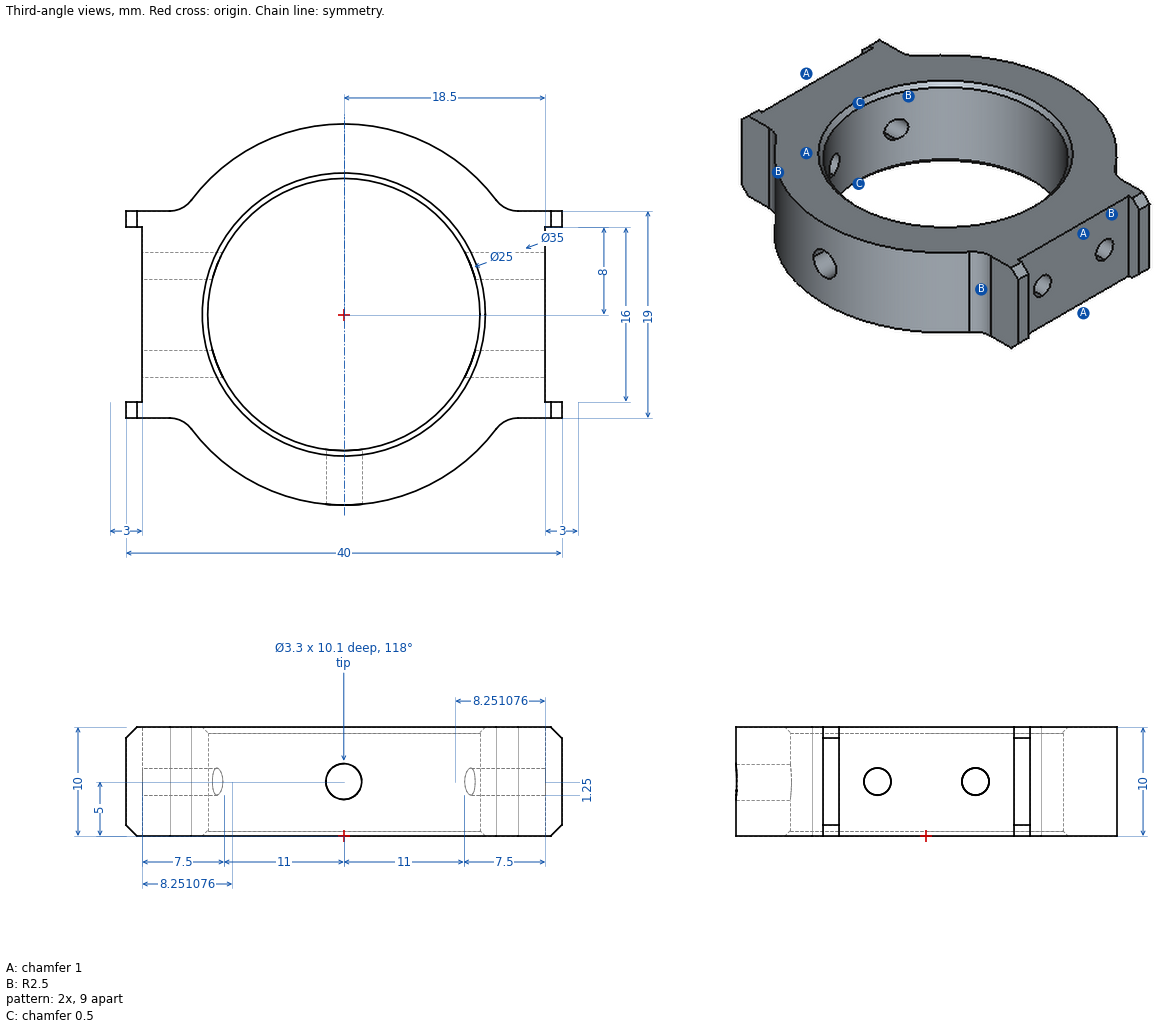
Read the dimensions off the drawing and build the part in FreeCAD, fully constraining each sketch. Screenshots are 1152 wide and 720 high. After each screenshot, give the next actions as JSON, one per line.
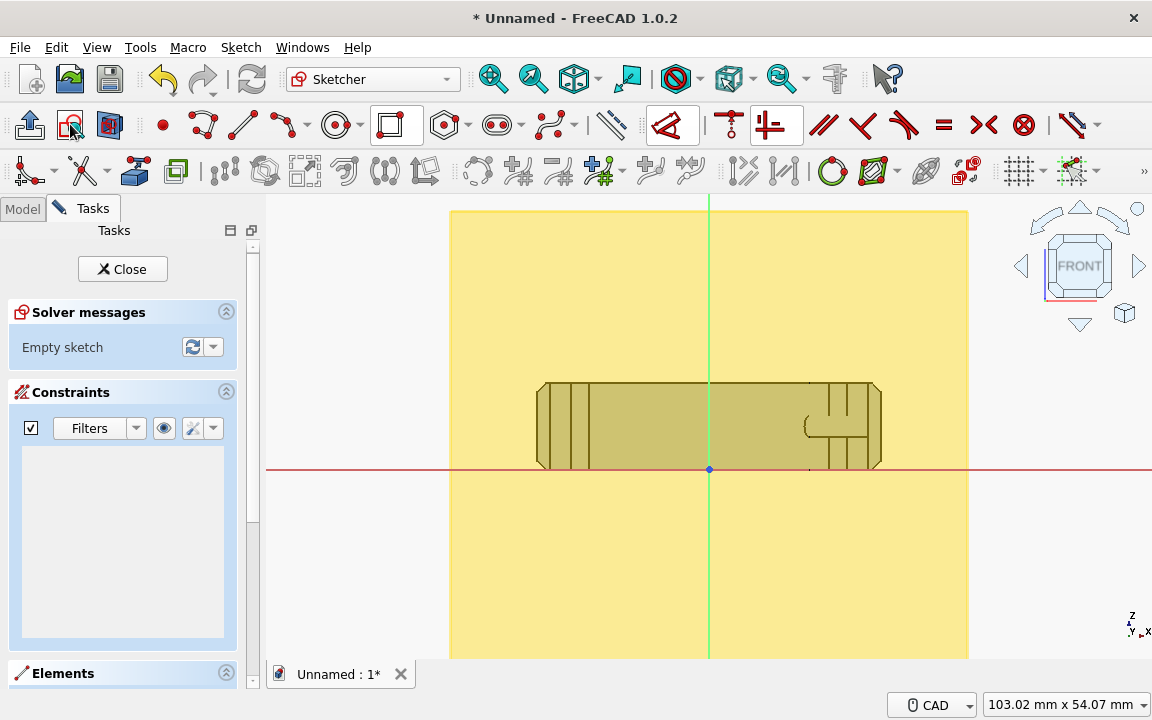
{"action": "scroll", "coordinate": [601, 461], "scroll_direction": "up", "scroll_amount": 5}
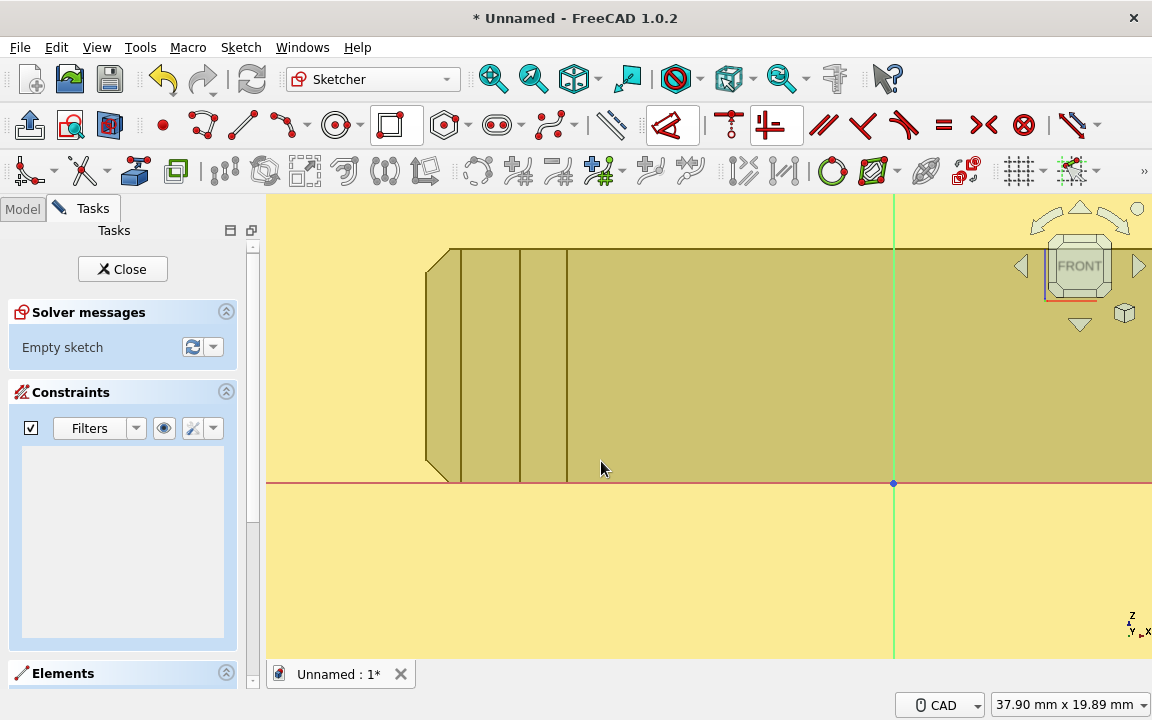
{"action": "left_click", "coordinate": [204, 126]}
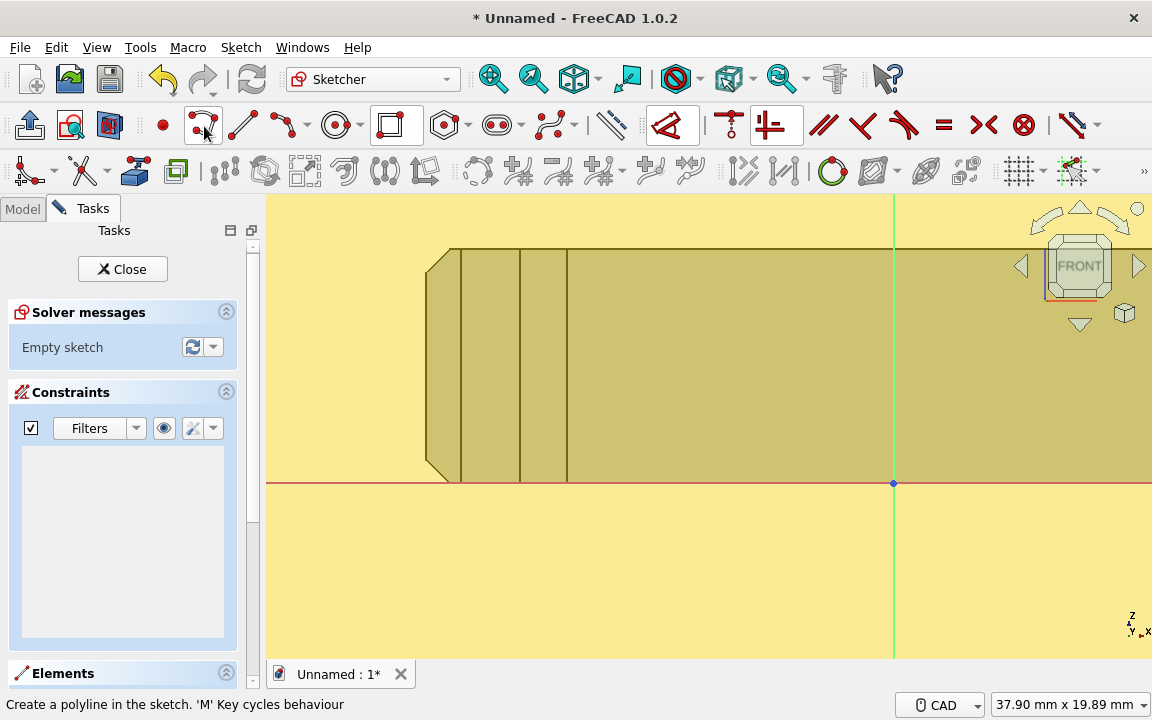
{"action": "left_click", "coordinate": [654, 366]}
{"action": "left_click", "coordinate": [637, 395]}
{"action": "left_click", "coordinate": [461, 395]}
{"action": "left_click", "coordinate": [461, 366]}
{"action": "left_click", "coordinate": [654, 367]}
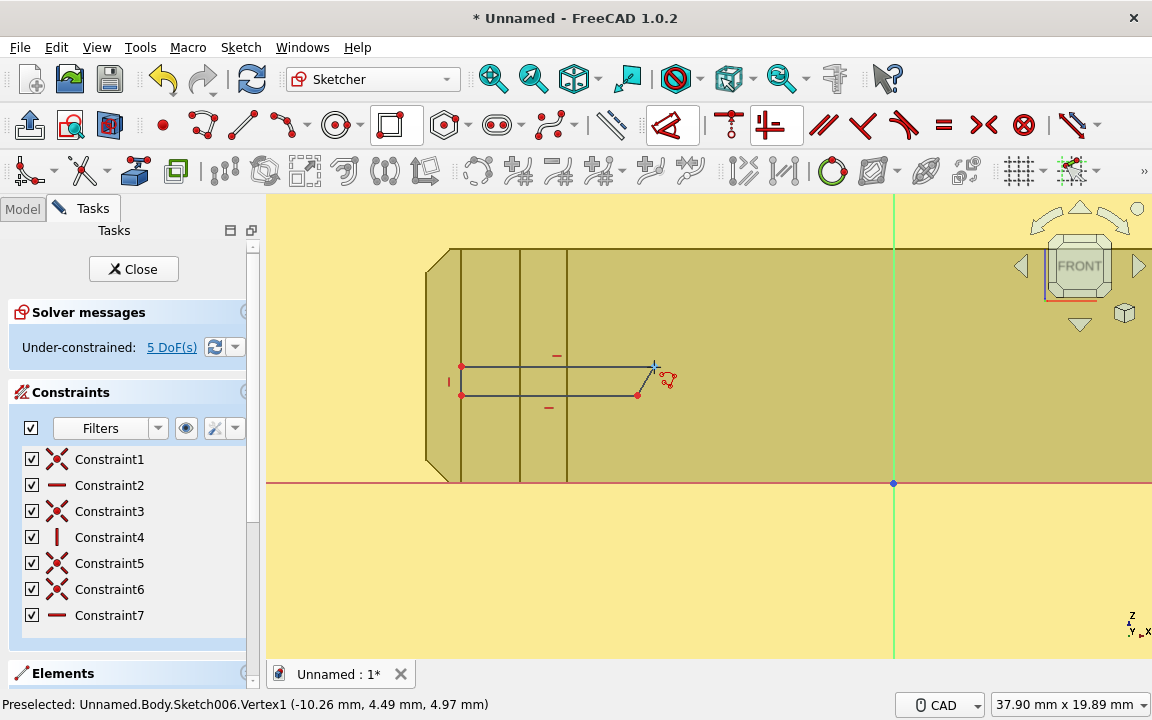
{"action": "left_click", "coordinate": [244, 126]}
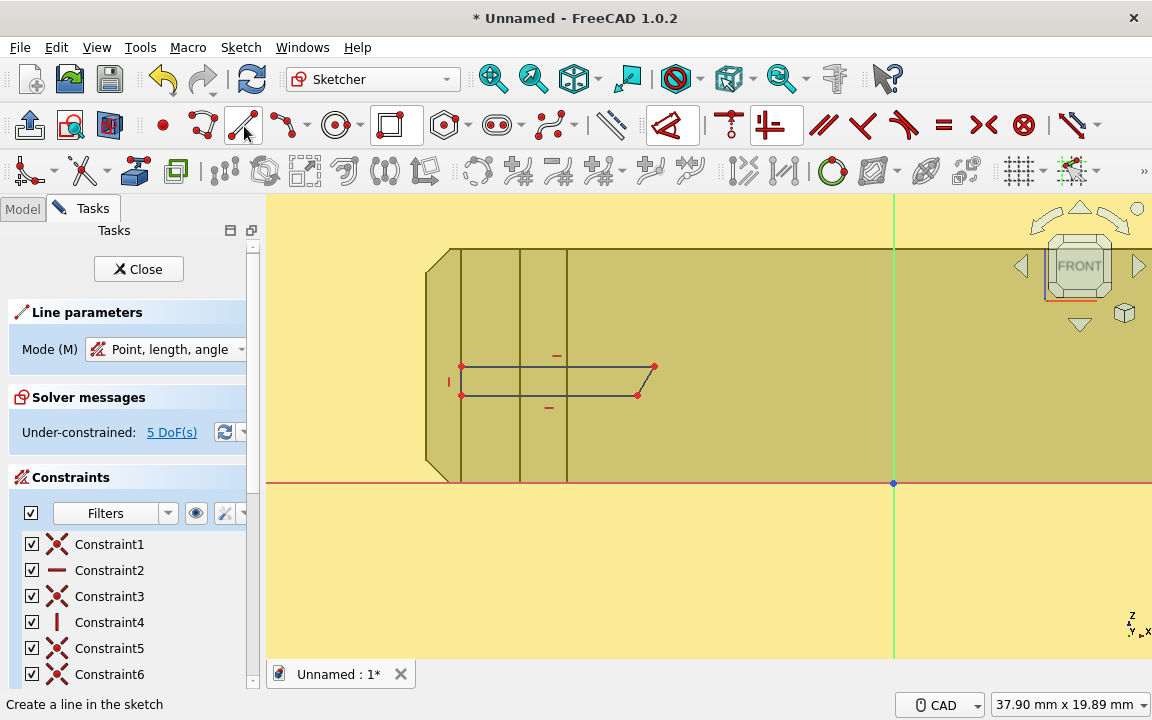
{"action": "left_click", "coordinate": [442, 366]}
{"action": "left_click", "coordinate": [384, 366]}
{"action": "key", "text": "Escape"}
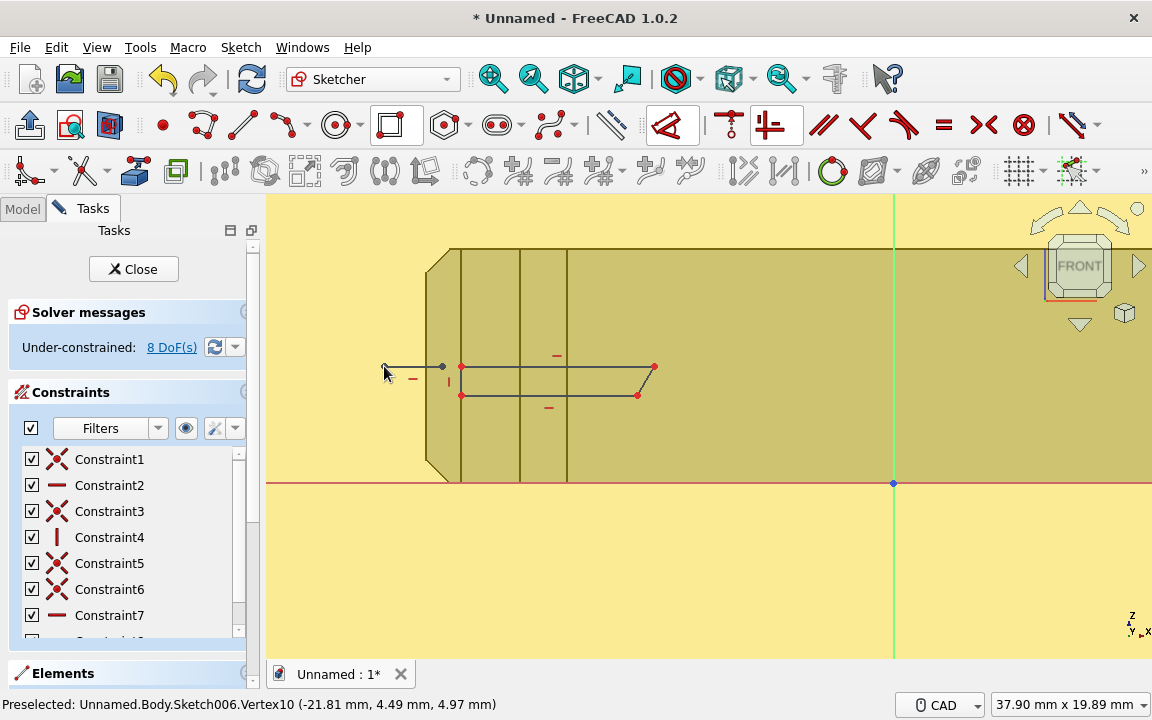
{"action": "left_click", "coordinate": [425, 367]}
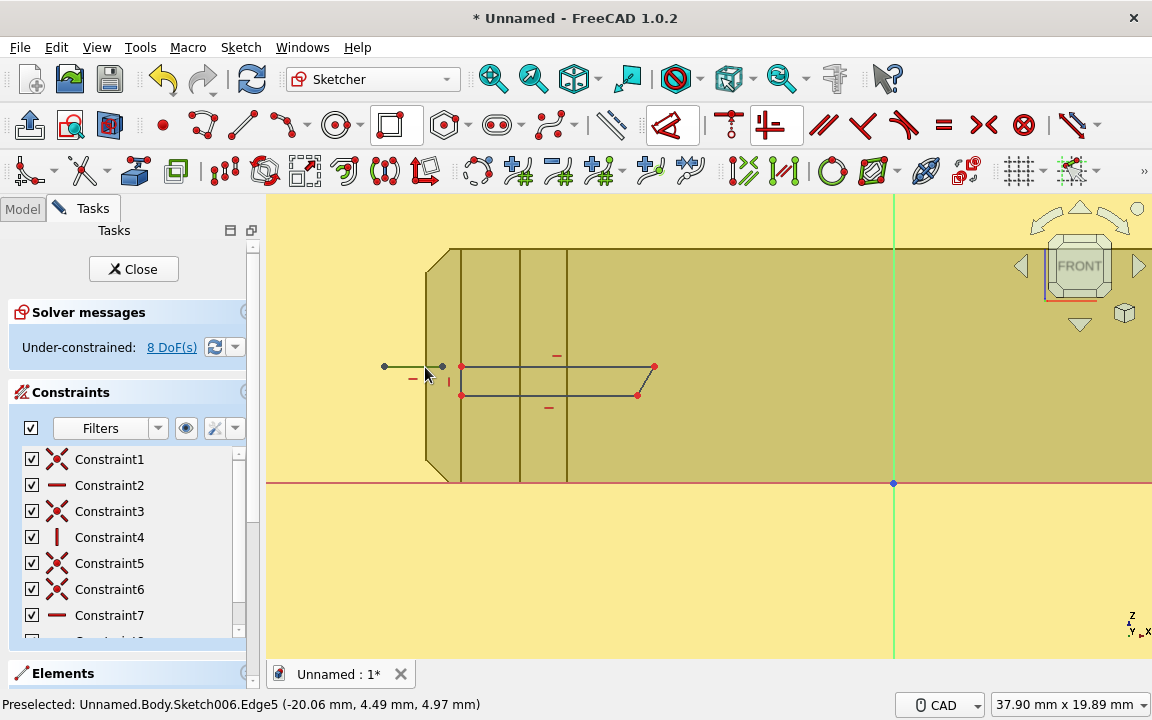
{"action": "key", "text": "g n"}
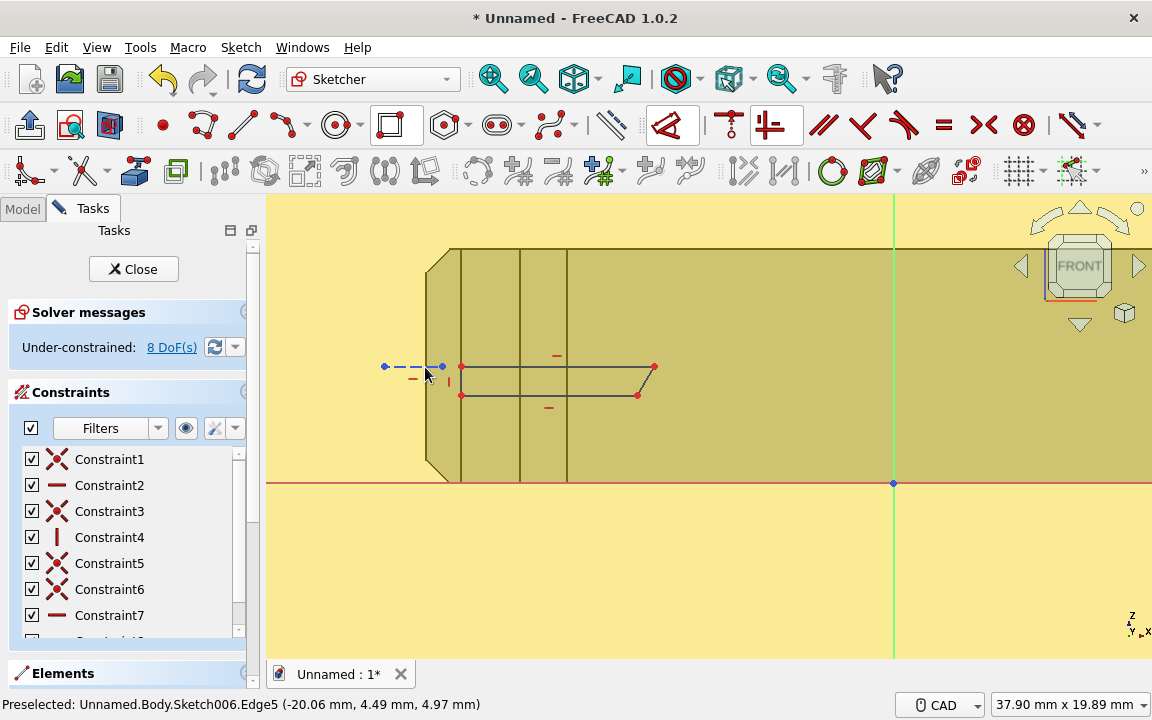
{"action": "left_click", "coordinate": [654, 367]}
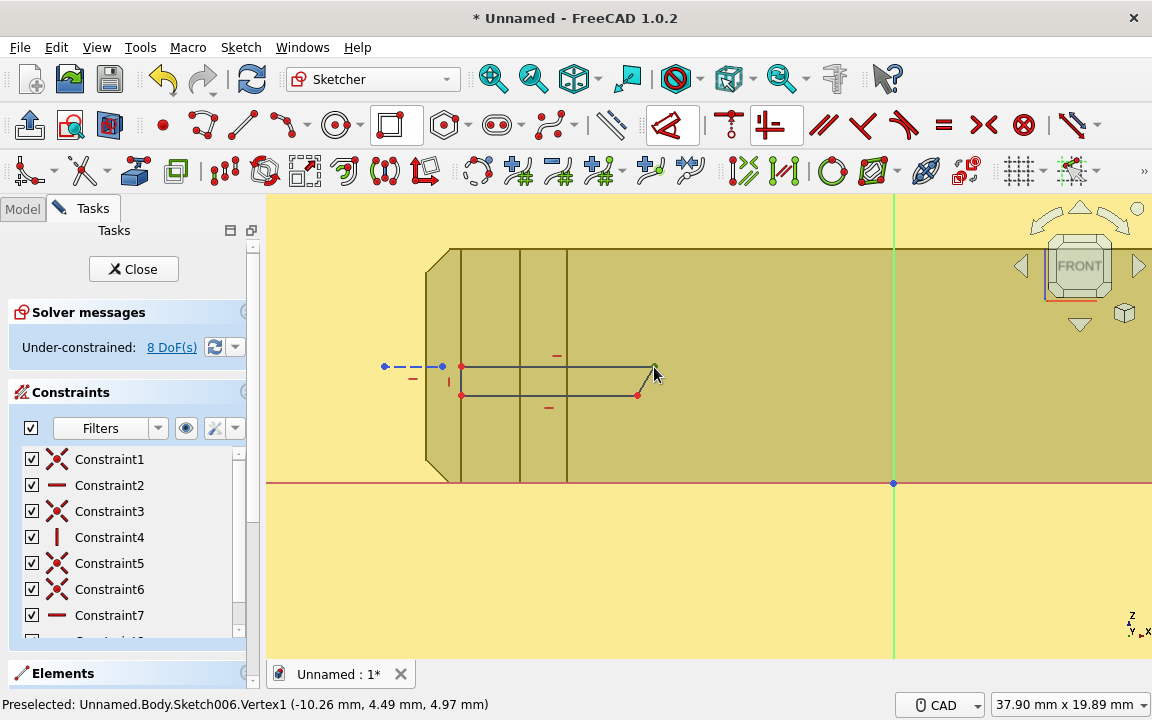
{"action": "key", "text": "i"}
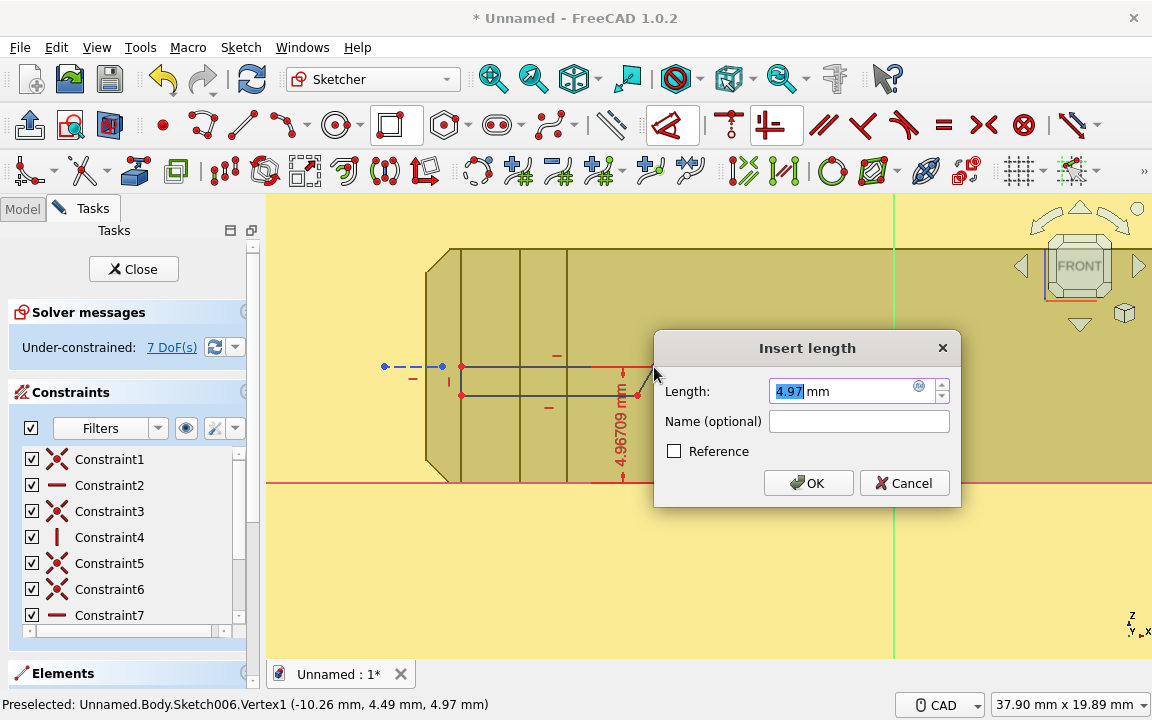
{"action": "type", "text": "5"}
{"action": "key", "text": "Return"}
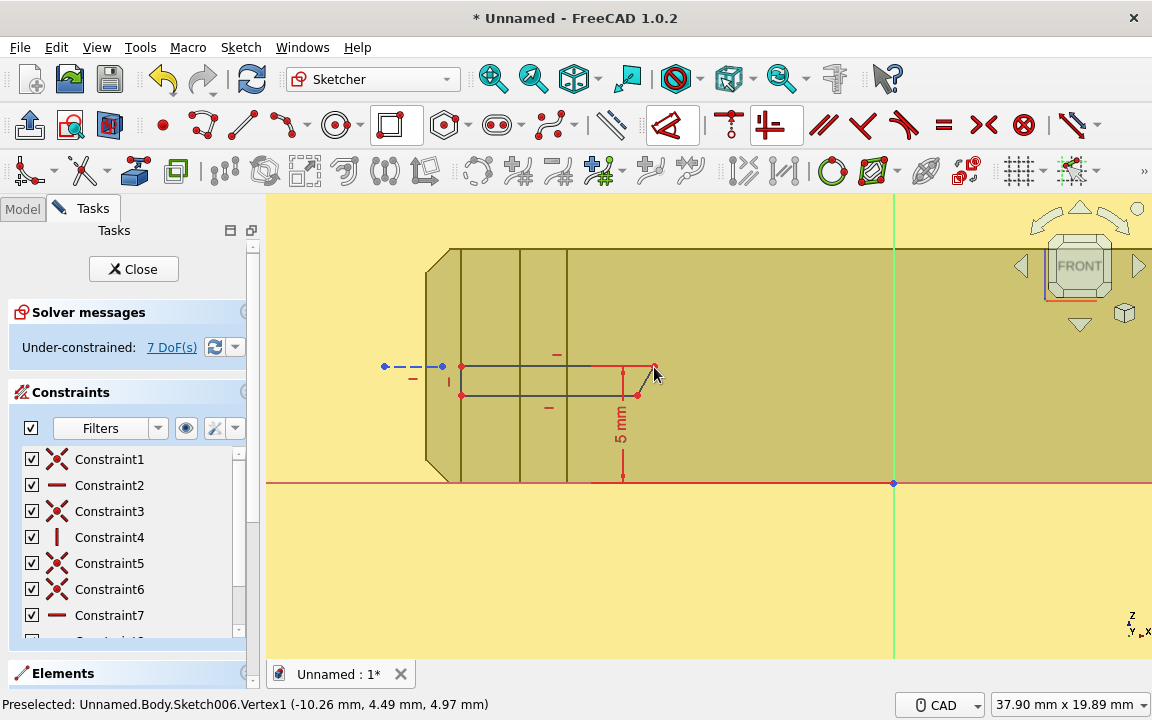
{"action": "left_click", "coordinate": [442, 367]}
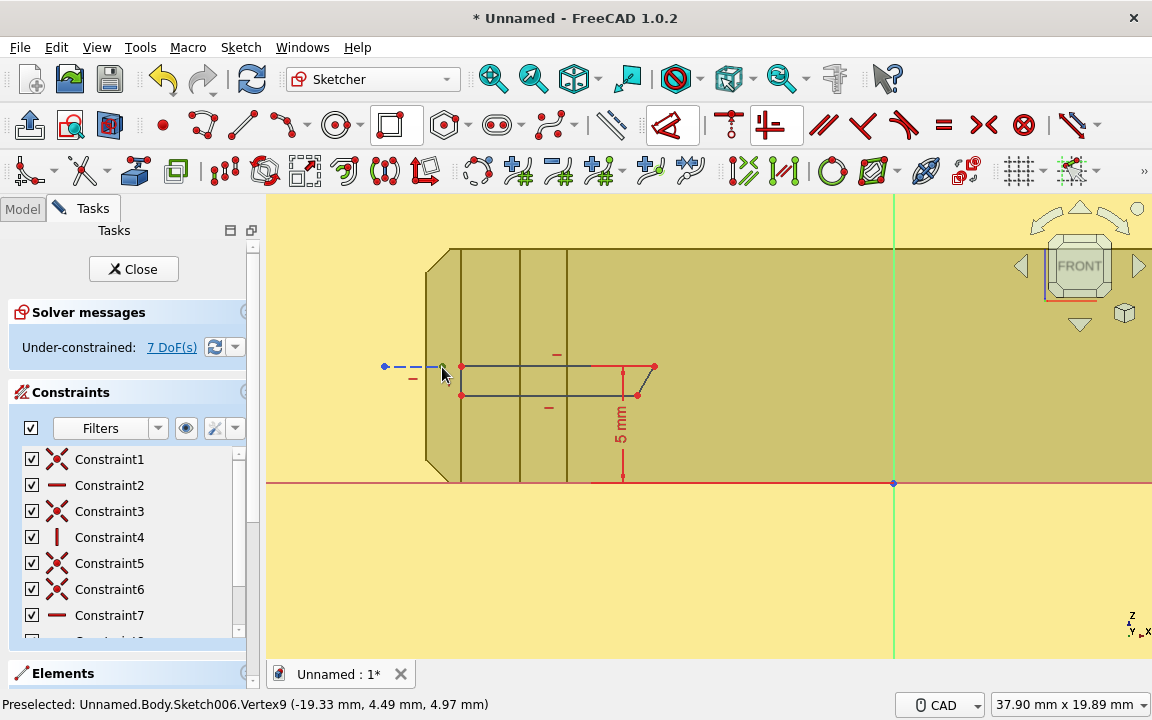
{"action": "key", "text": "i"}